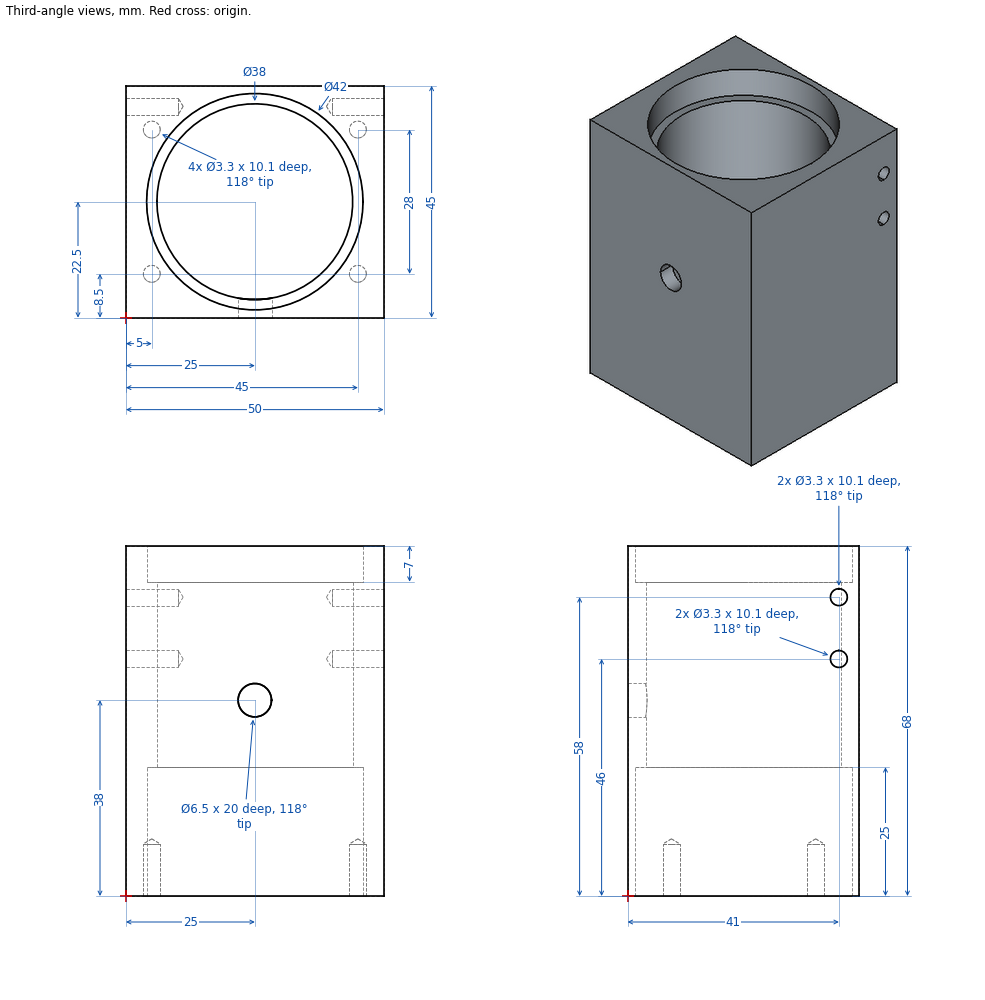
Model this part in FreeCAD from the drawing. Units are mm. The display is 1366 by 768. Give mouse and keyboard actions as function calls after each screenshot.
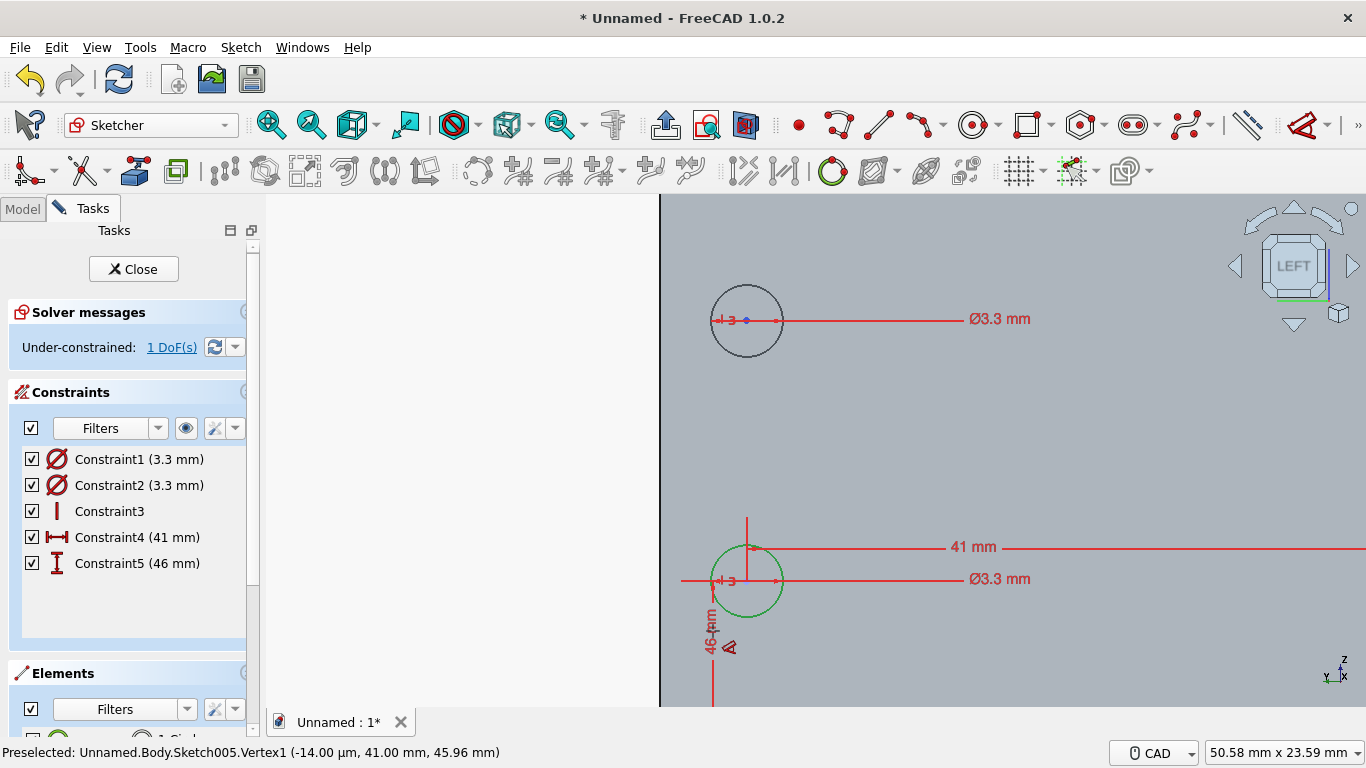
click(747, 321)
click(713, 500)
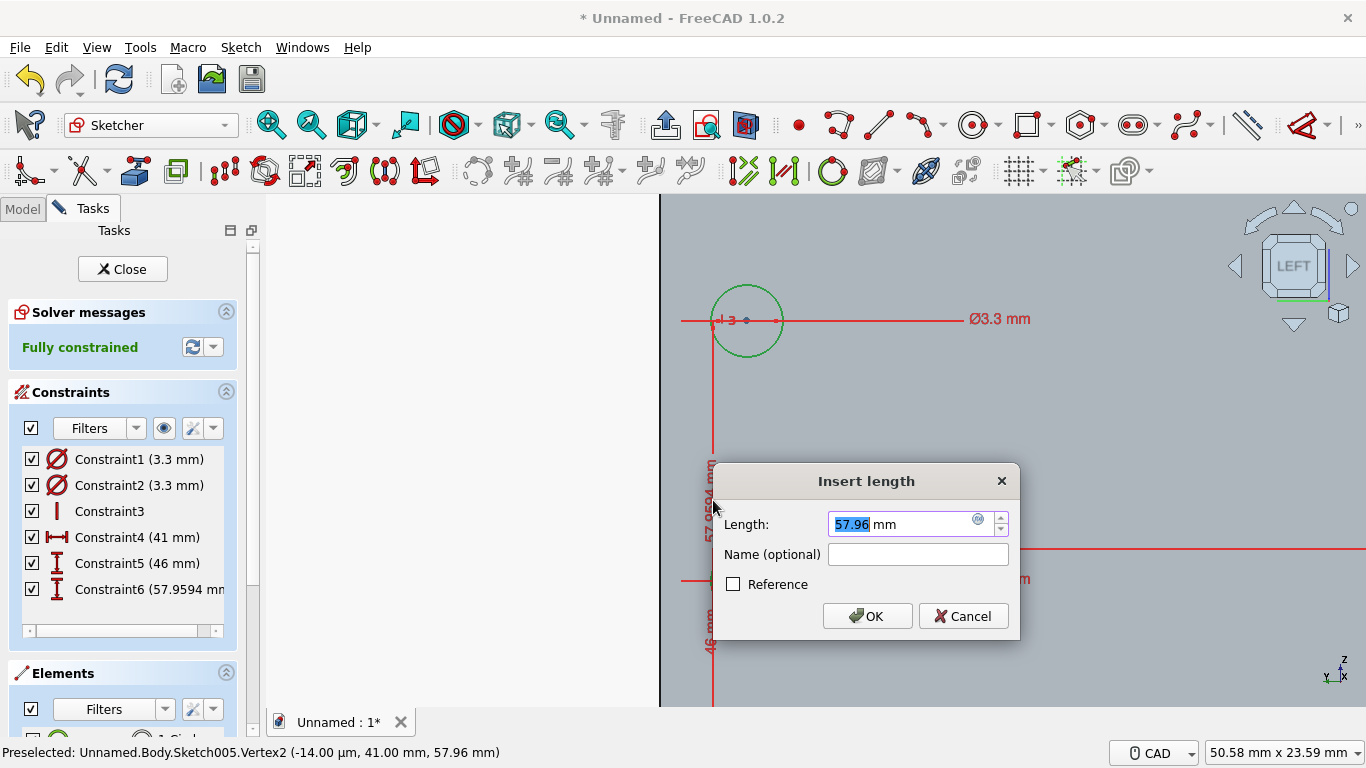
text(58)
key(Return)
key(Escape)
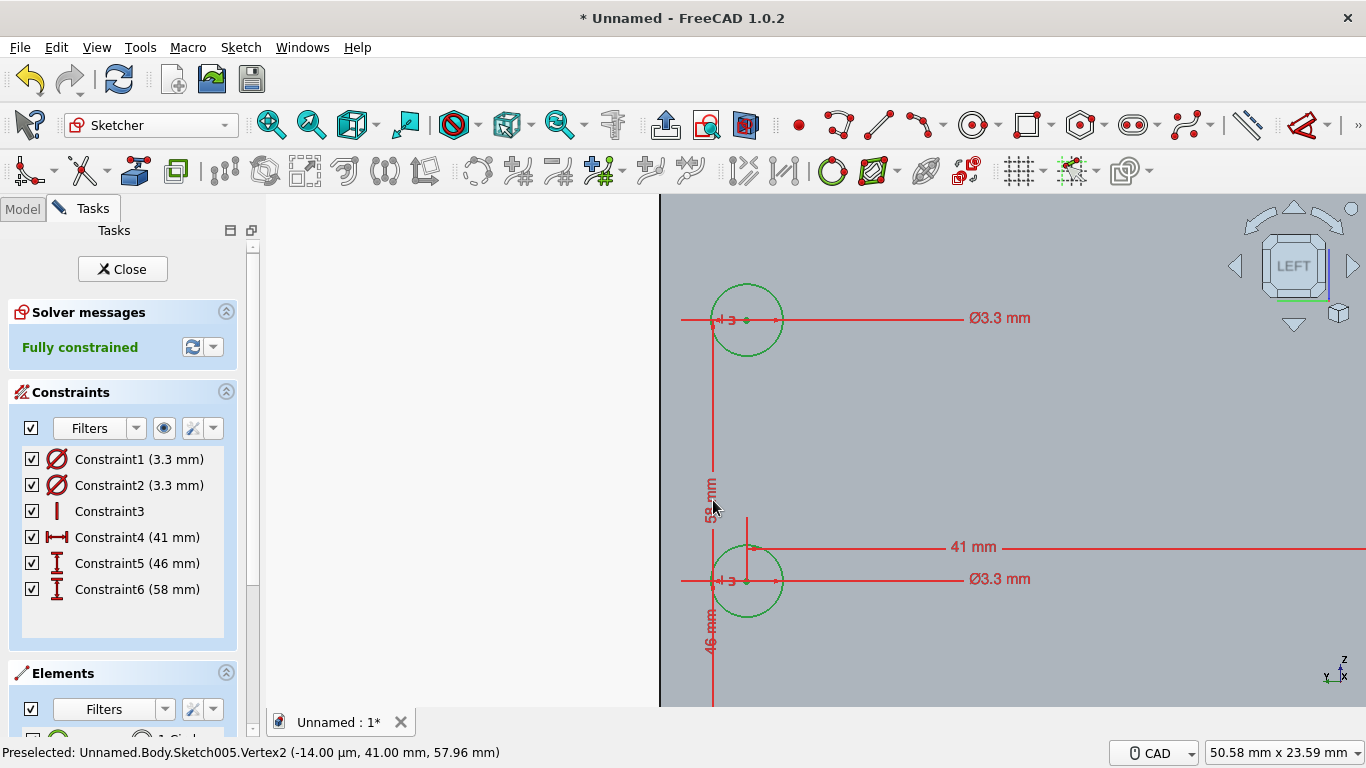
click(123, 269)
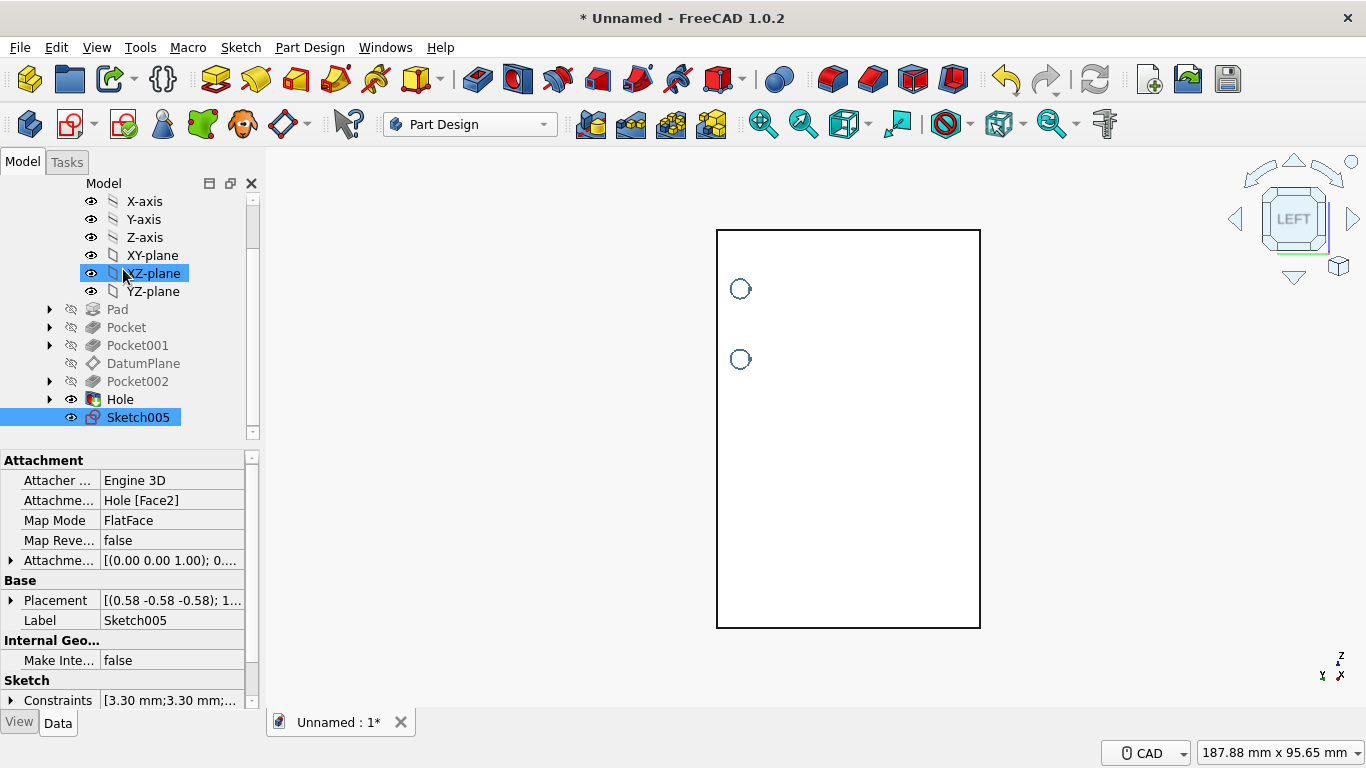
click(518, 80)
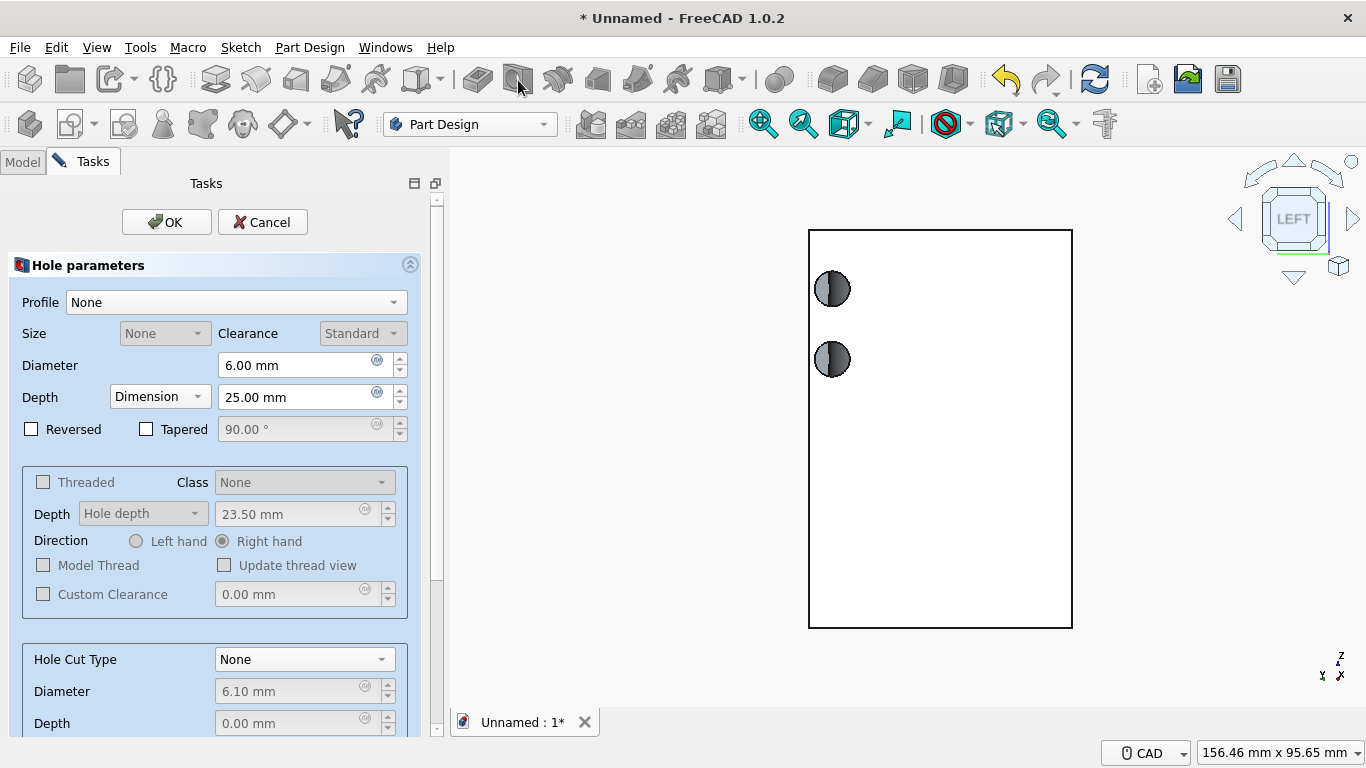
triple_click(305, 365)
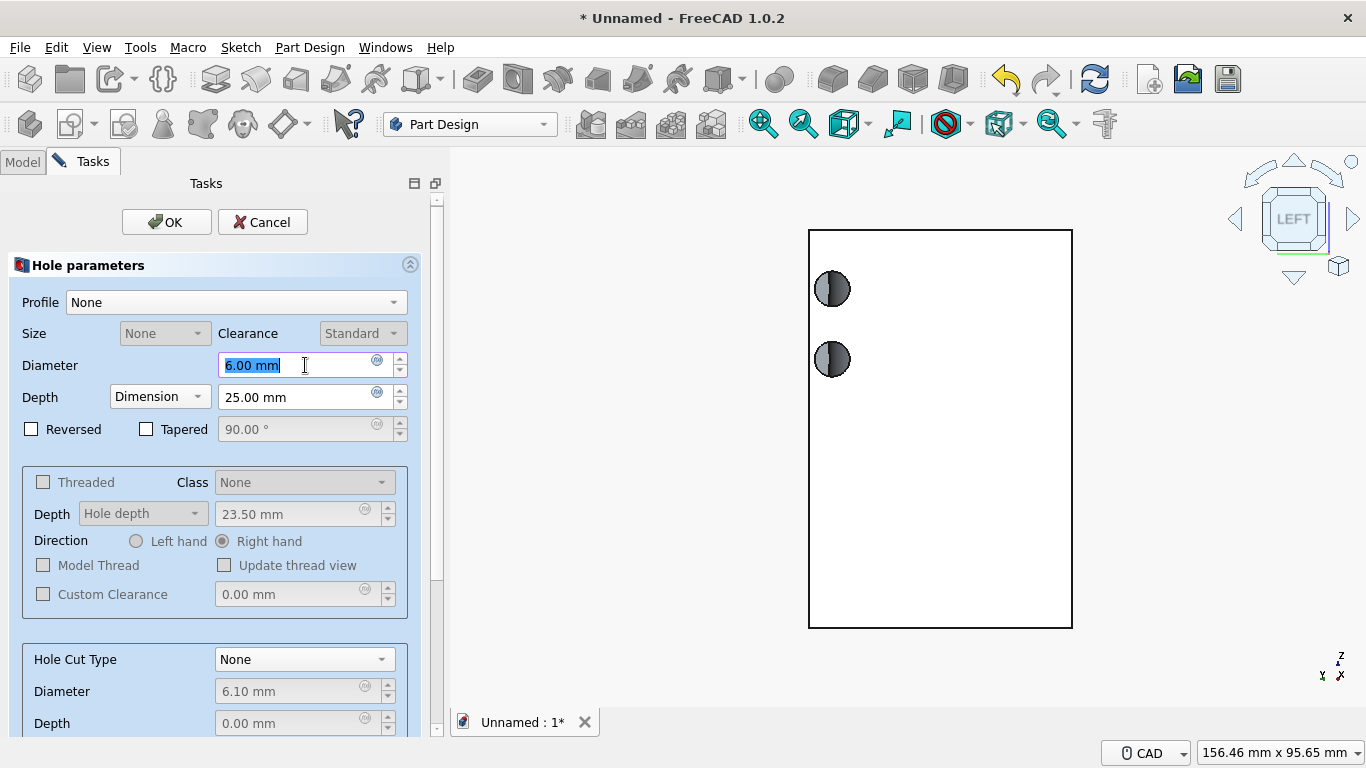
text(3.3)
key(Tab)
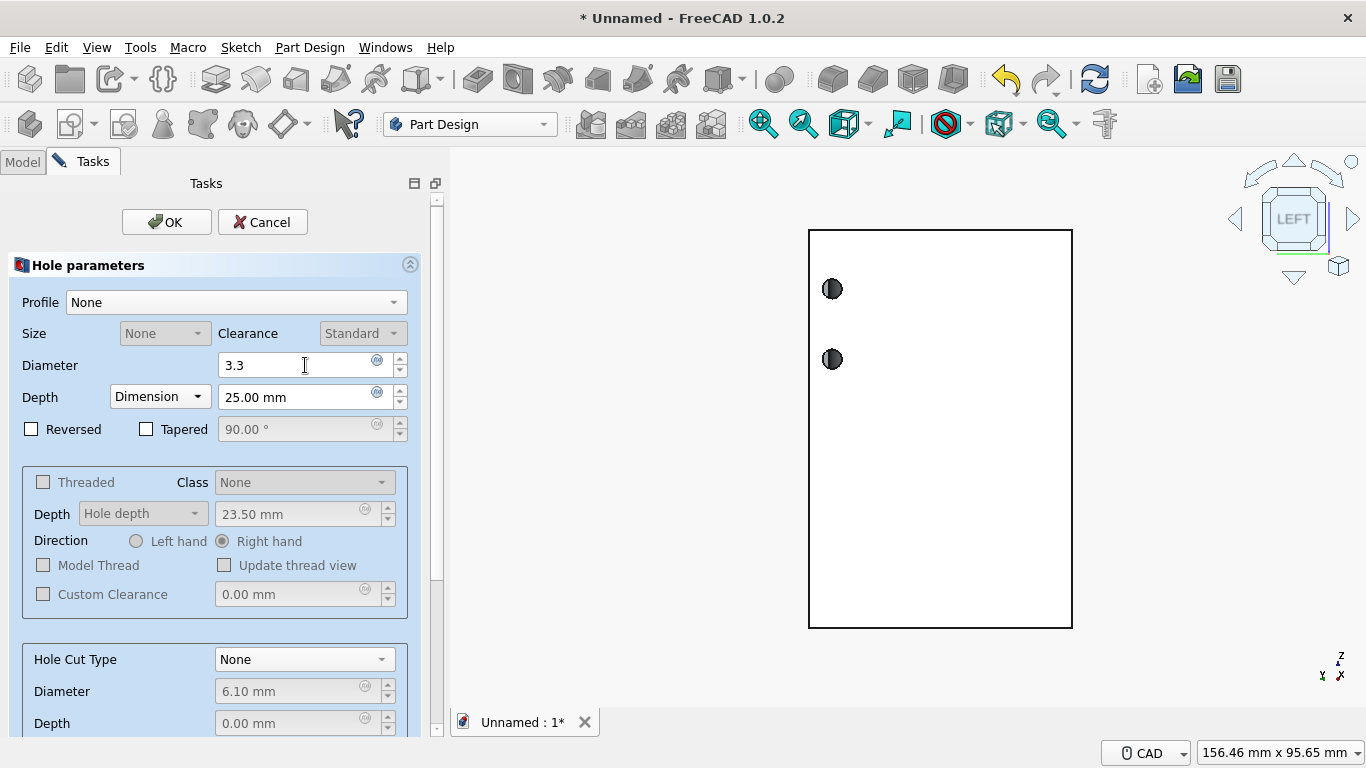
triple_click(305, 397)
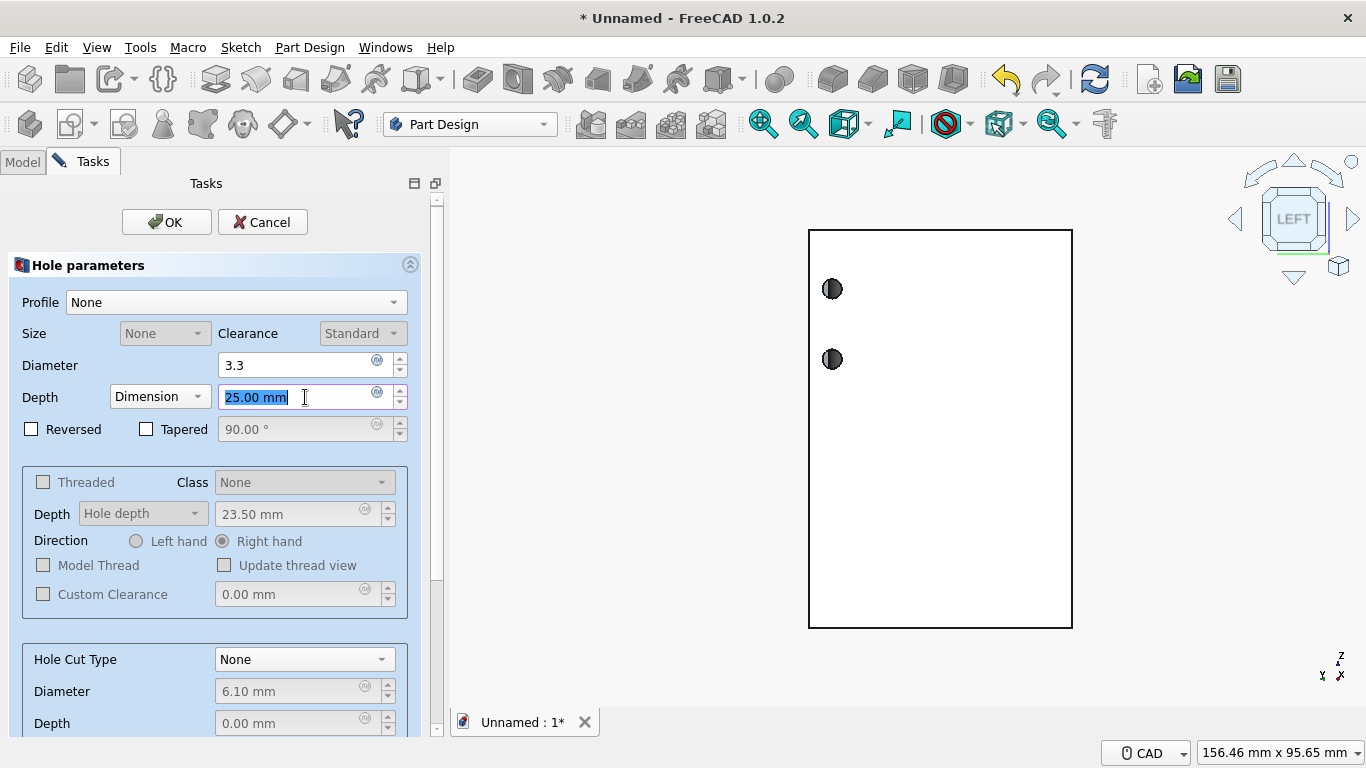
text(10.1)
key(Tab)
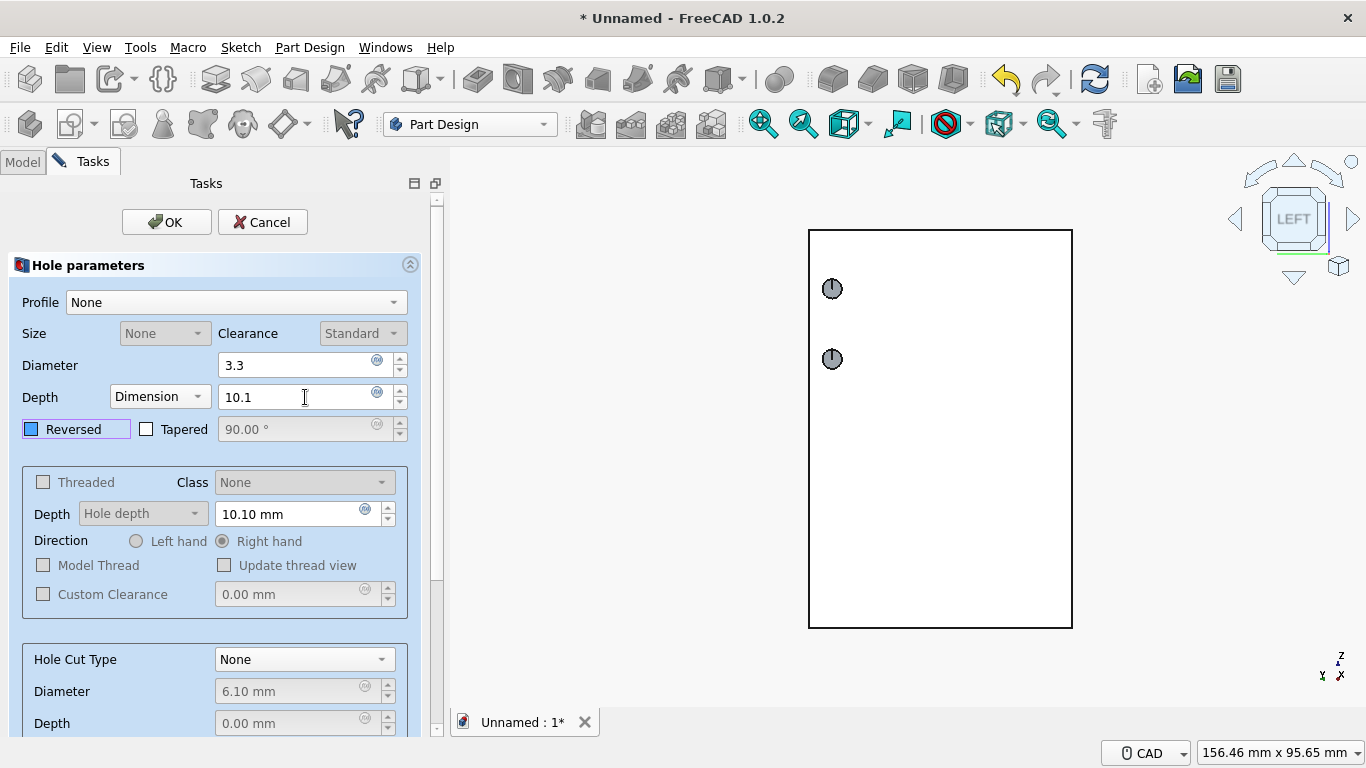
click(167, 222)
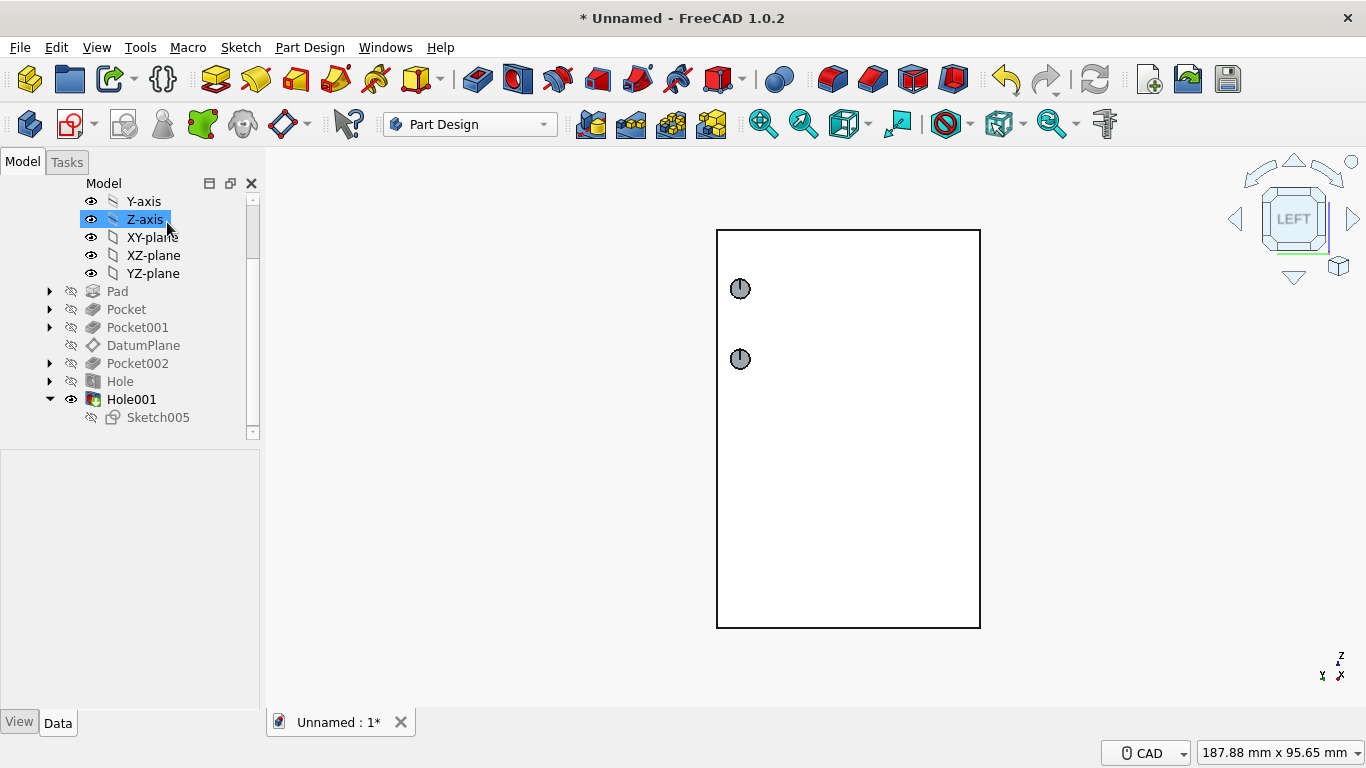
click(70, 124)